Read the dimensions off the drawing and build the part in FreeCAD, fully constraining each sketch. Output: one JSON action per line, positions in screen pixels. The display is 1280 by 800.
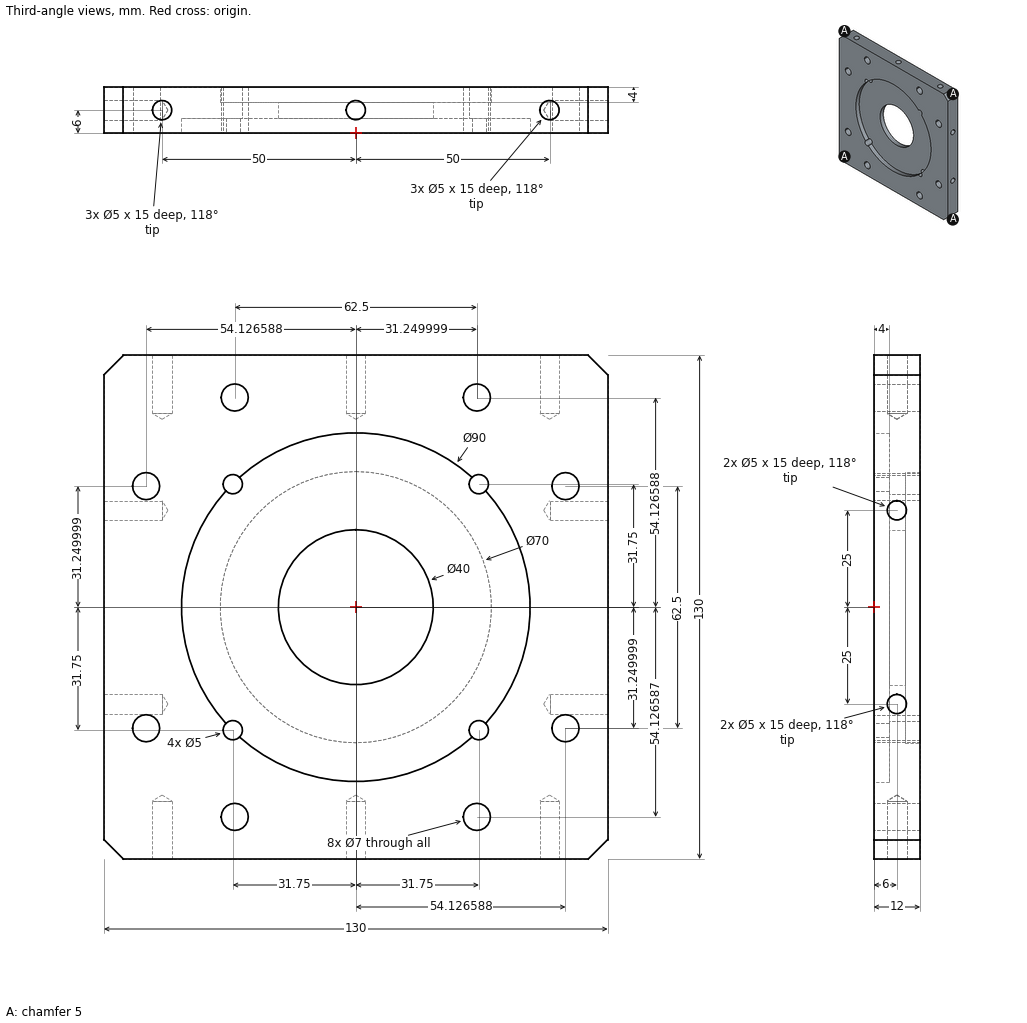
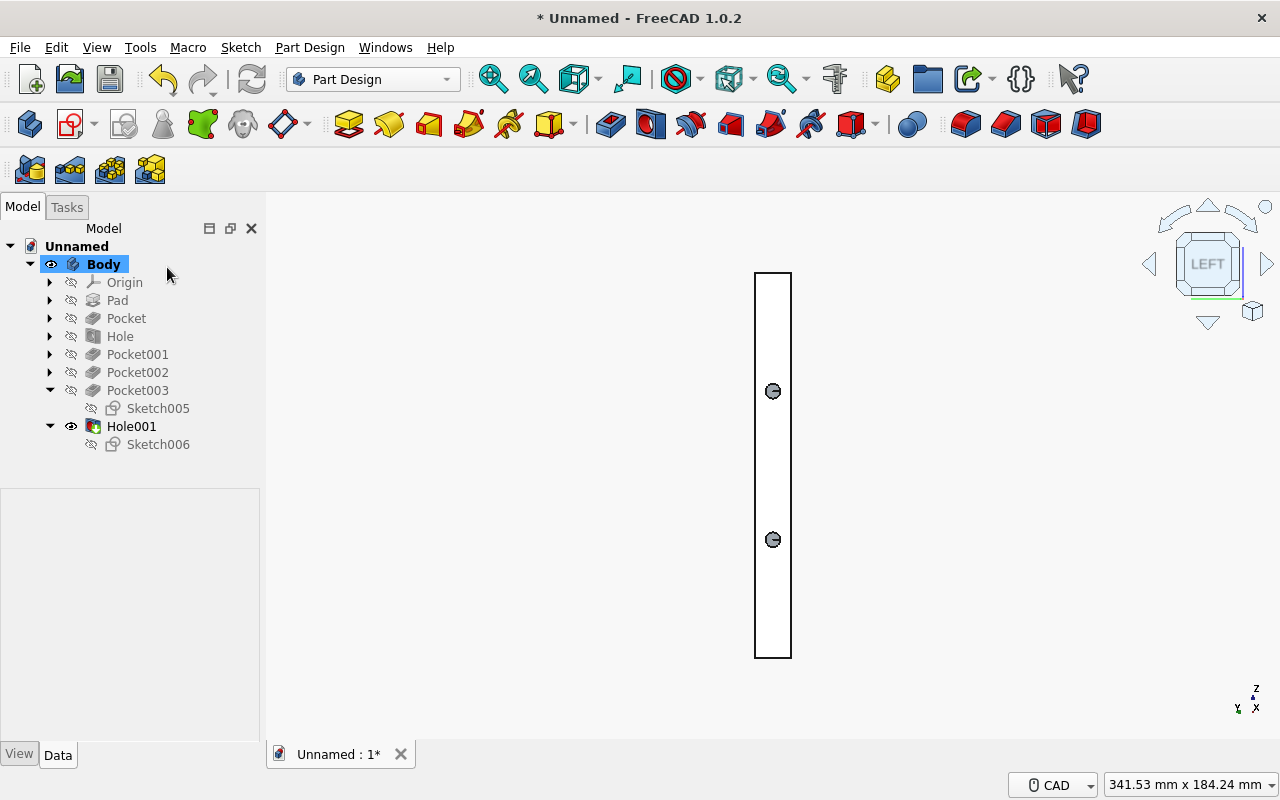
{"action": "key", "text": "0"}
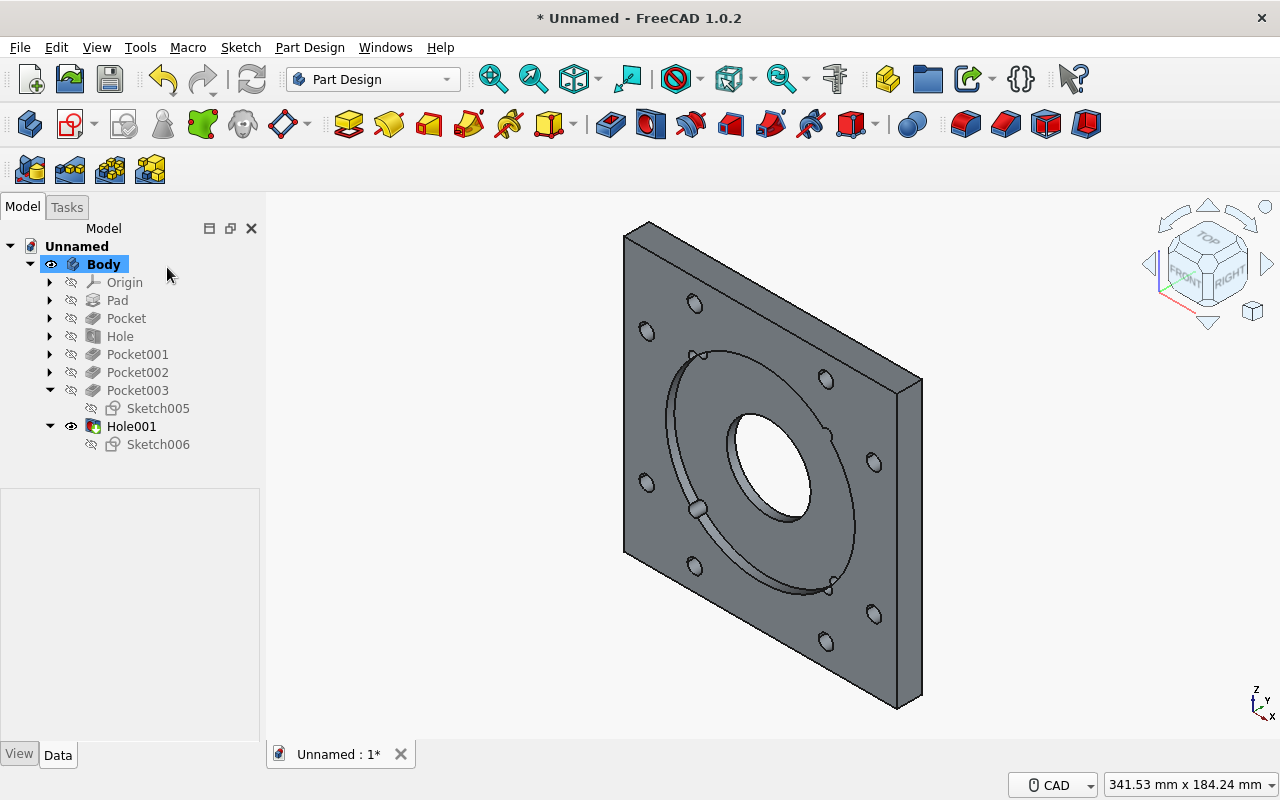
{"action": "left_click", "coordinate": [909, 453]}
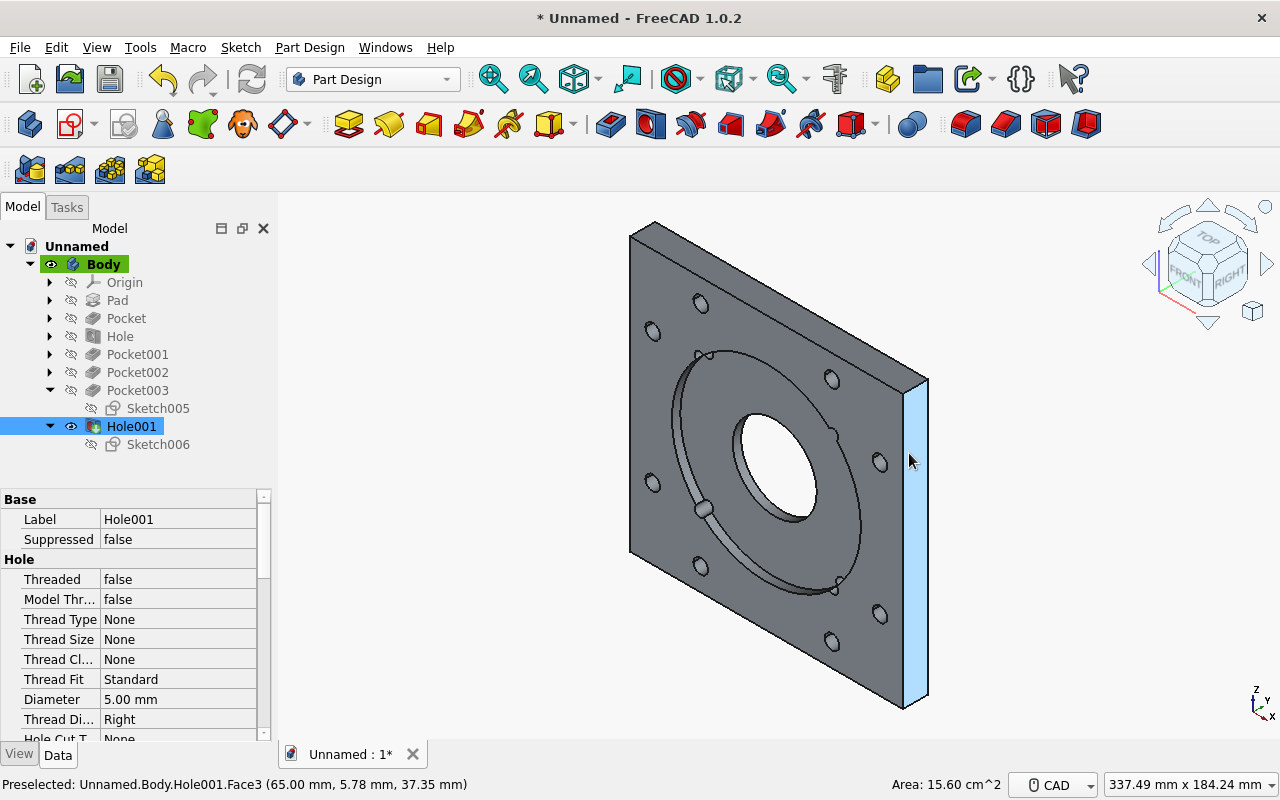
{"action": "left_click", "coordinate": [70, 124]}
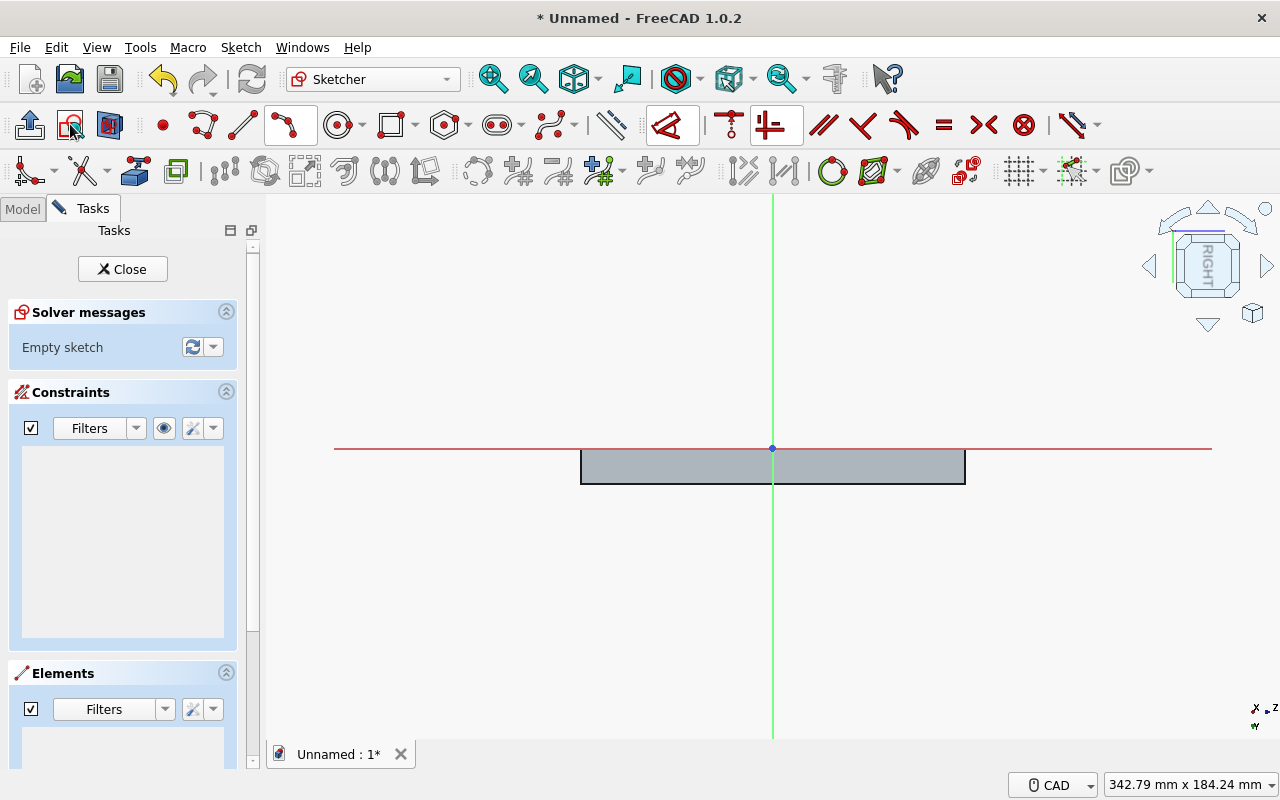
{"action": "scroll", "coordinate": [803, 459], "scroll_direction": "up", "scroll_amount": 6}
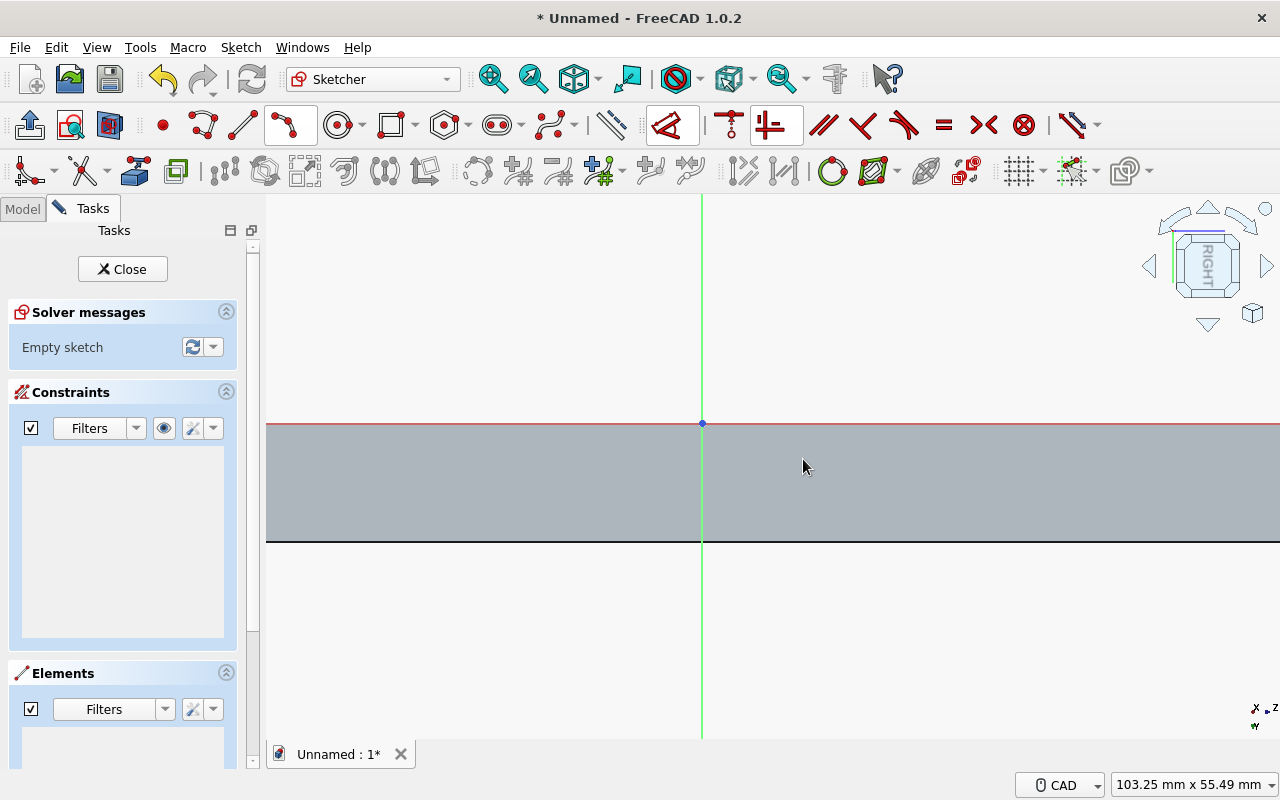
{"action": "left_click", "coordinate": [338, 126]}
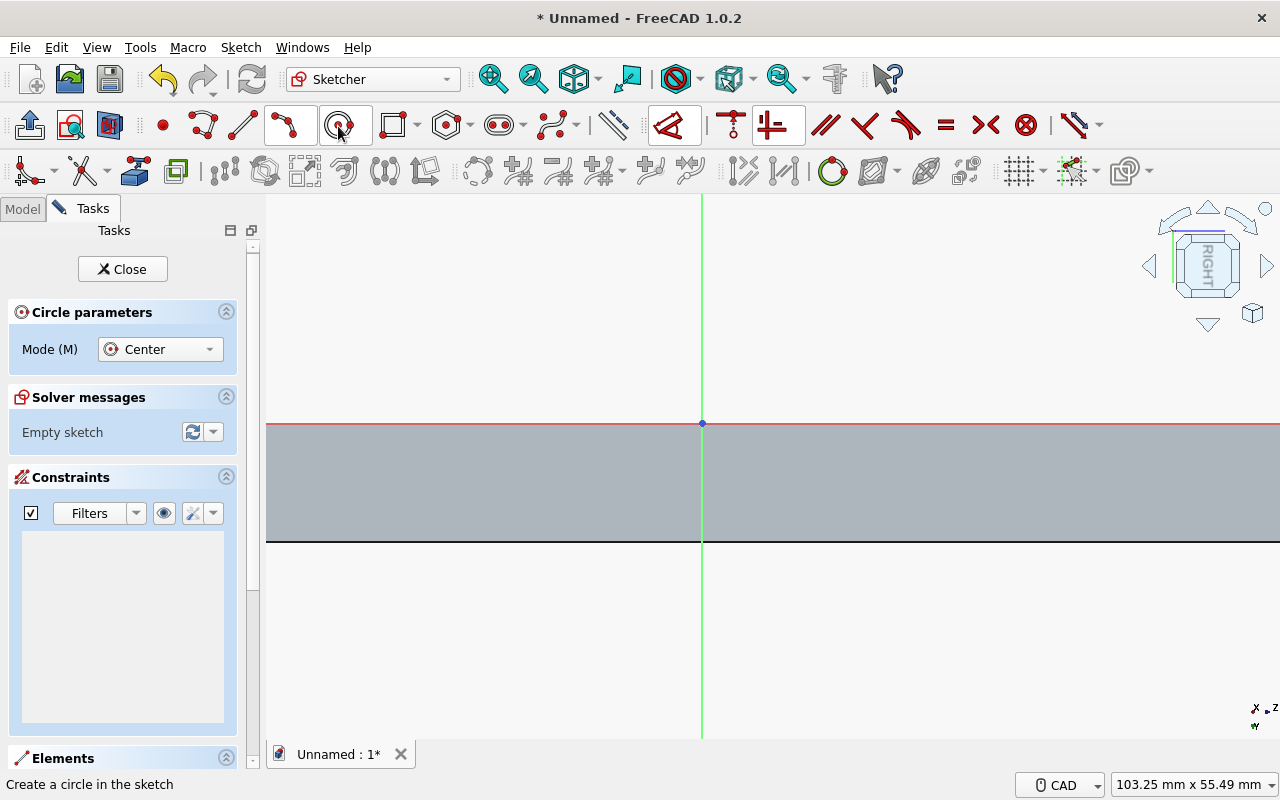
{"action": "left_click", "coordinate": [948, 483]}
{"action": "left_click", "coordinate": [965, 465]}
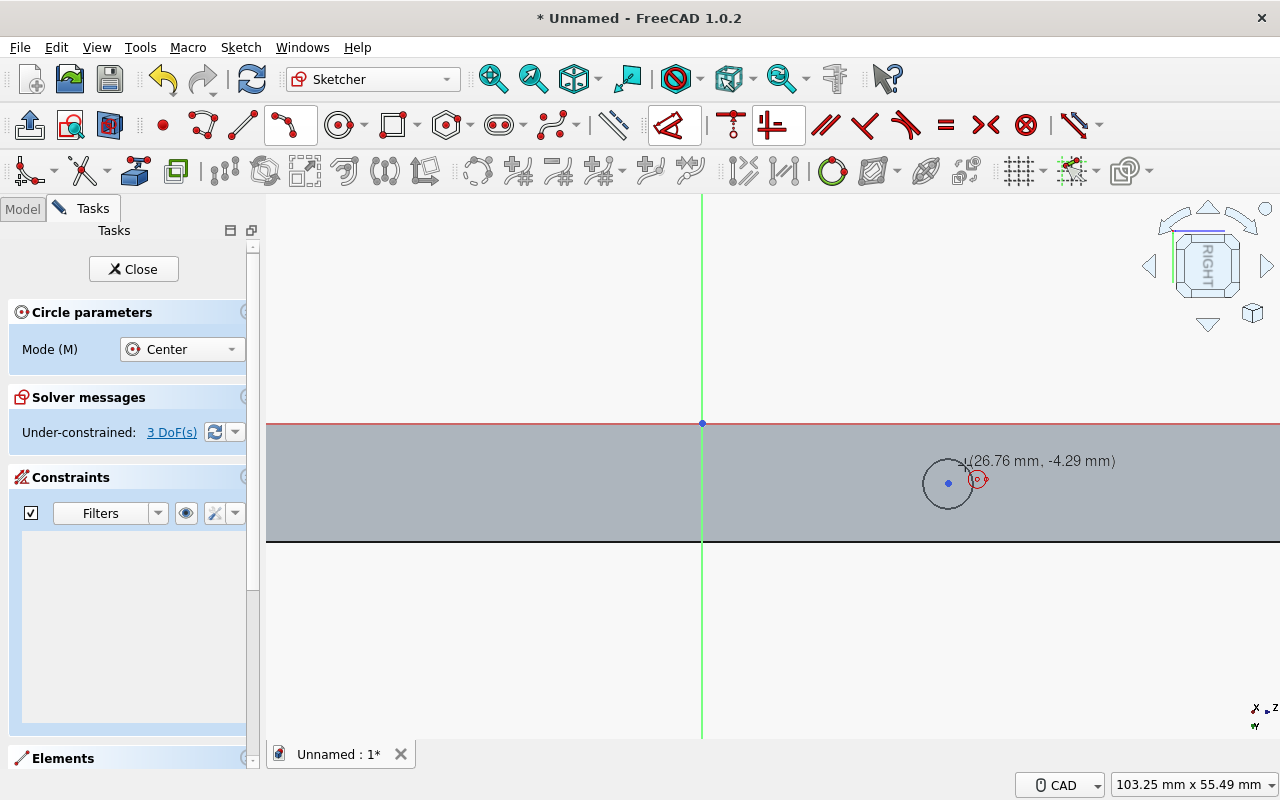
{"action": "left_click", "coordinate": [457, 483]}
{"action": "left_click", "coordinate": [474, 465]}
{"action": "key", "text": "Escape"}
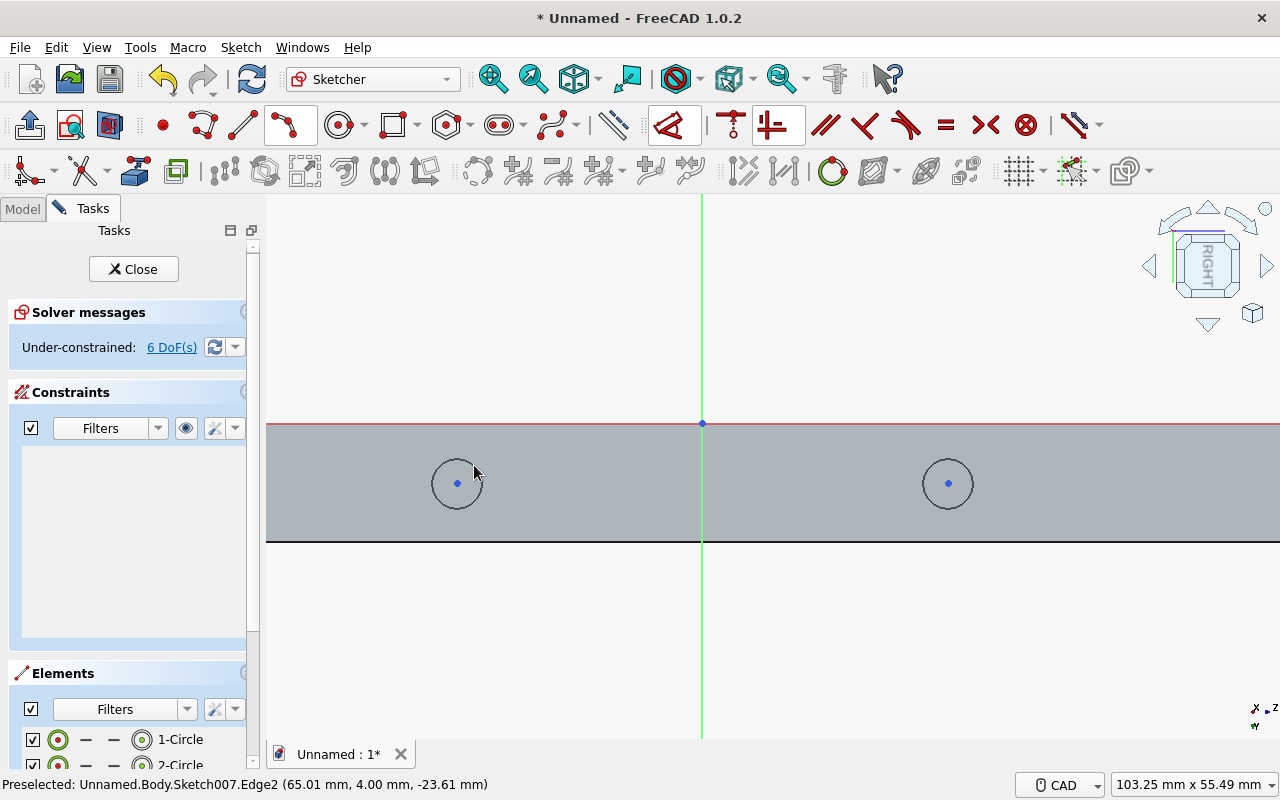
{"action": "left_click", "coordinate": [965, 466]}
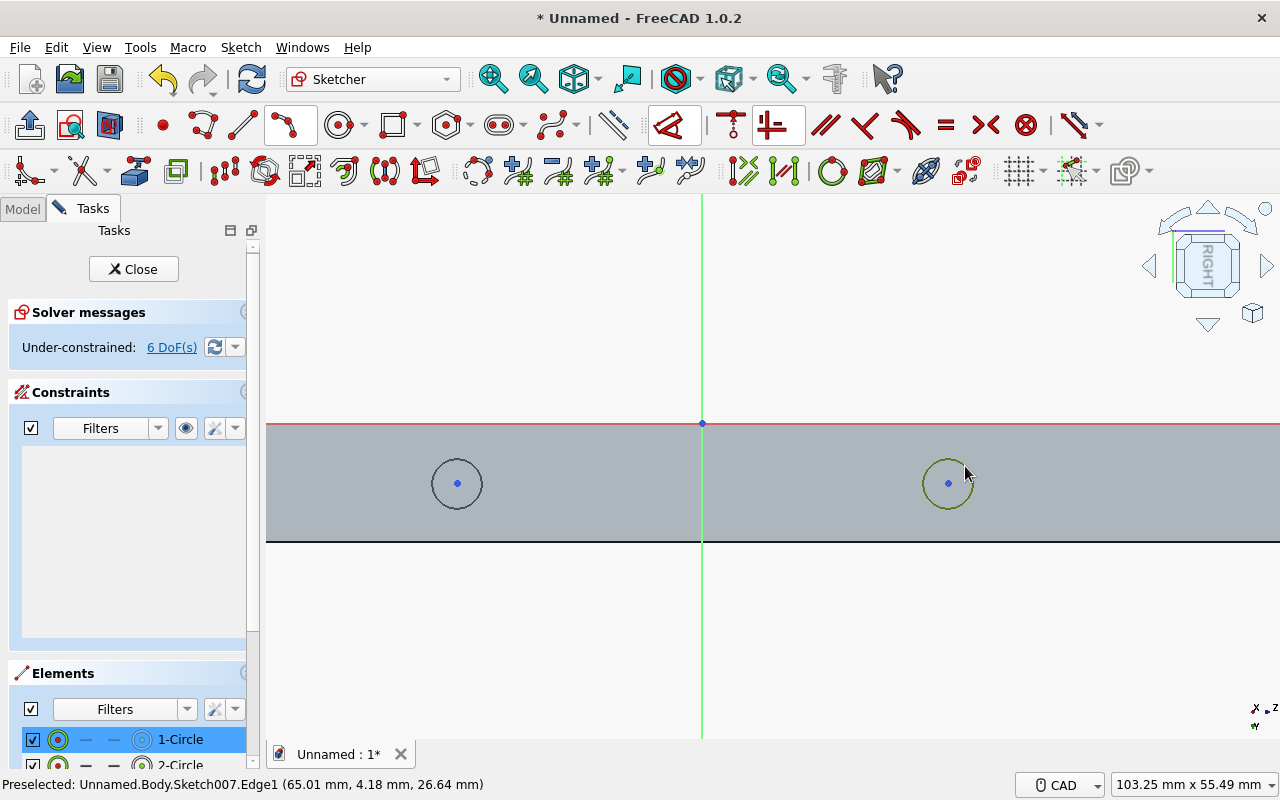
{"action": "left_click", "coordinate": [474, 466]}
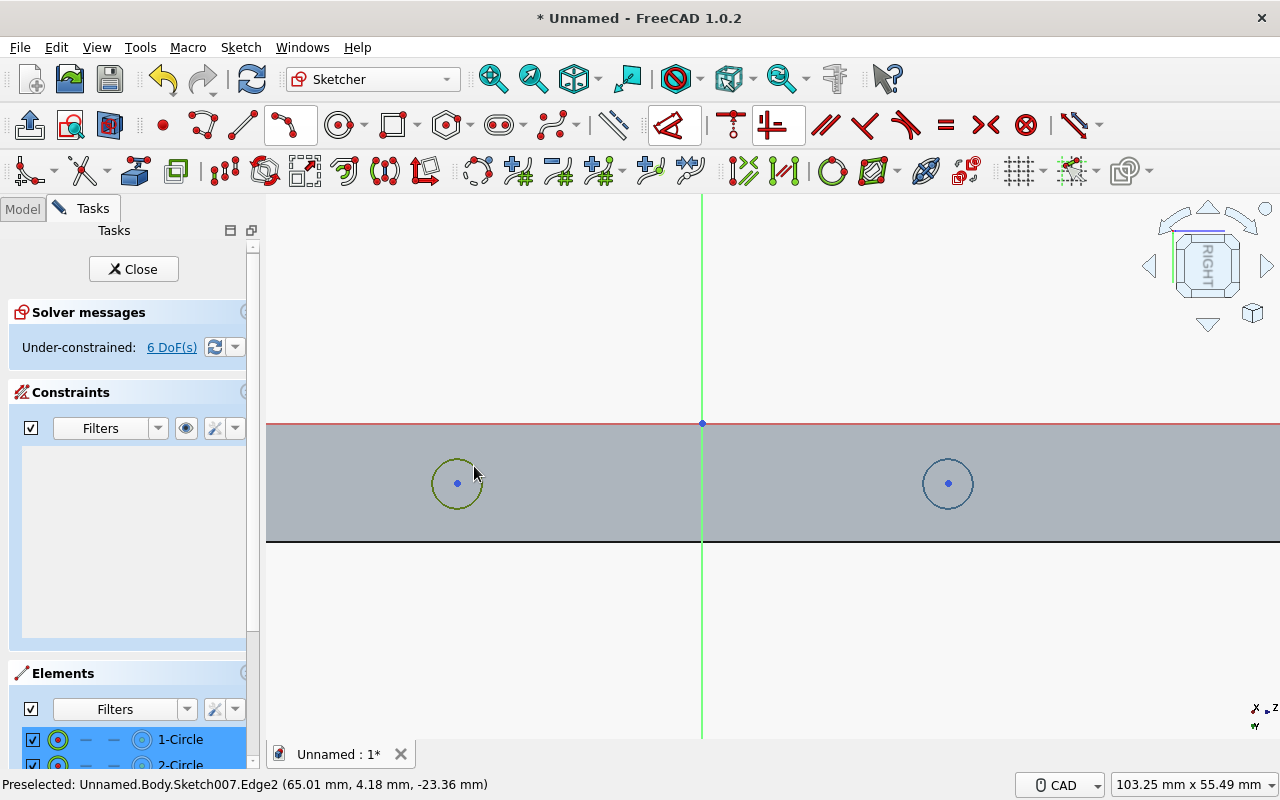
{"action": "key", "text": "e"}